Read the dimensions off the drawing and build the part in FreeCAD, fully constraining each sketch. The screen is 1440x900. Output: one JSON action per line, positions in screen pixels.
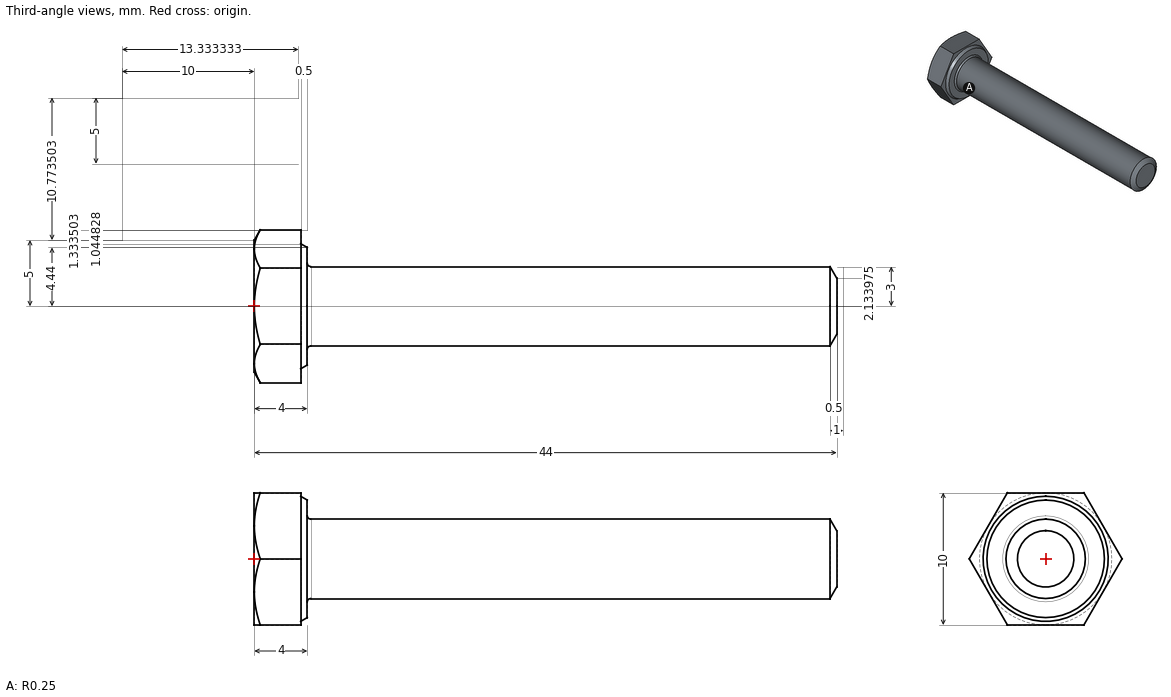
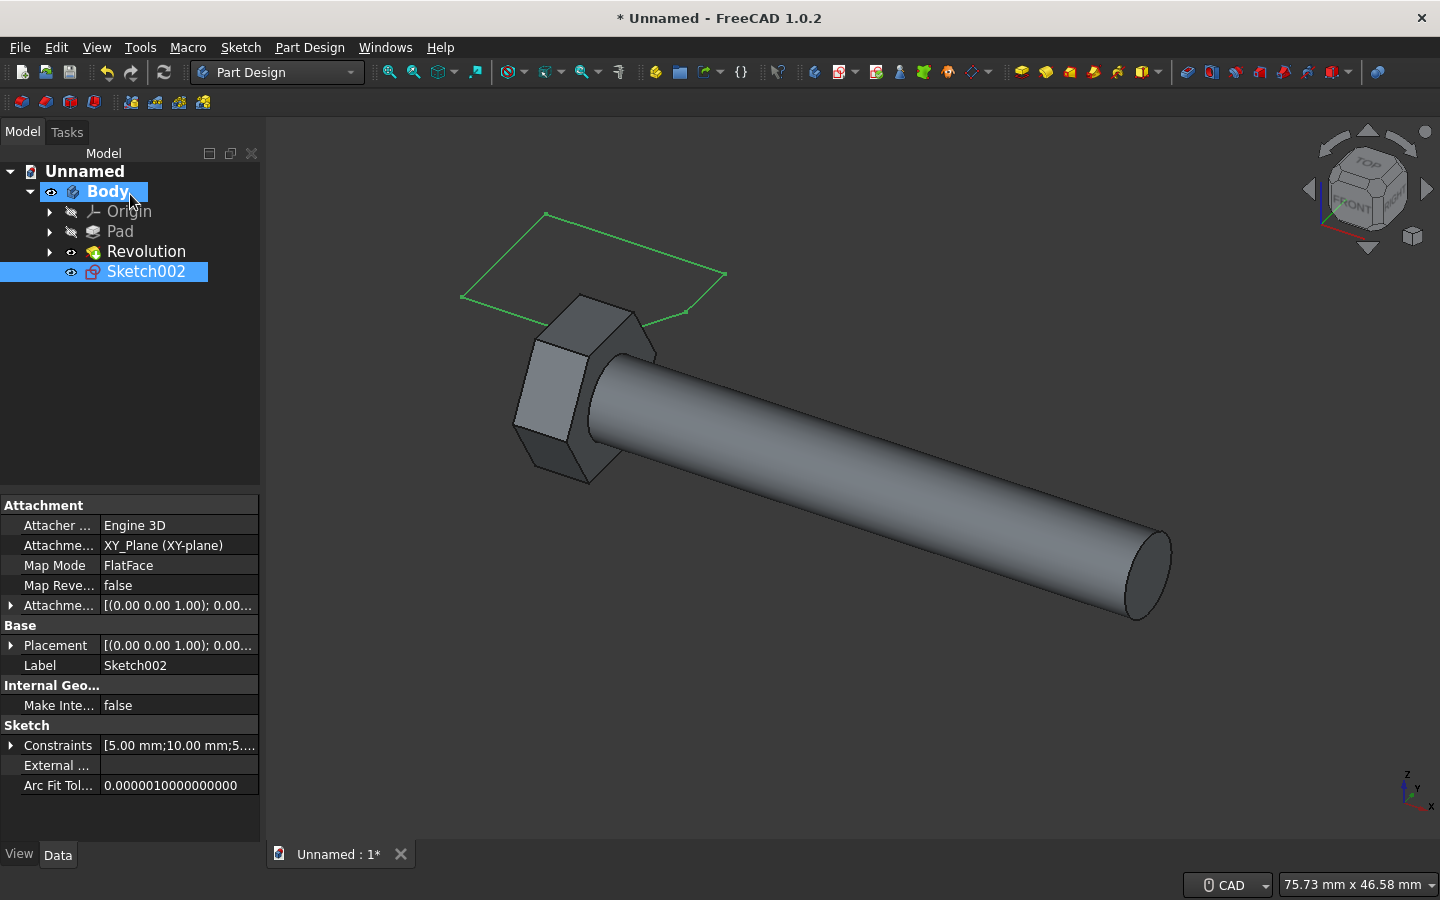
{"action": "left_click", "coordinate": [1236, 72]}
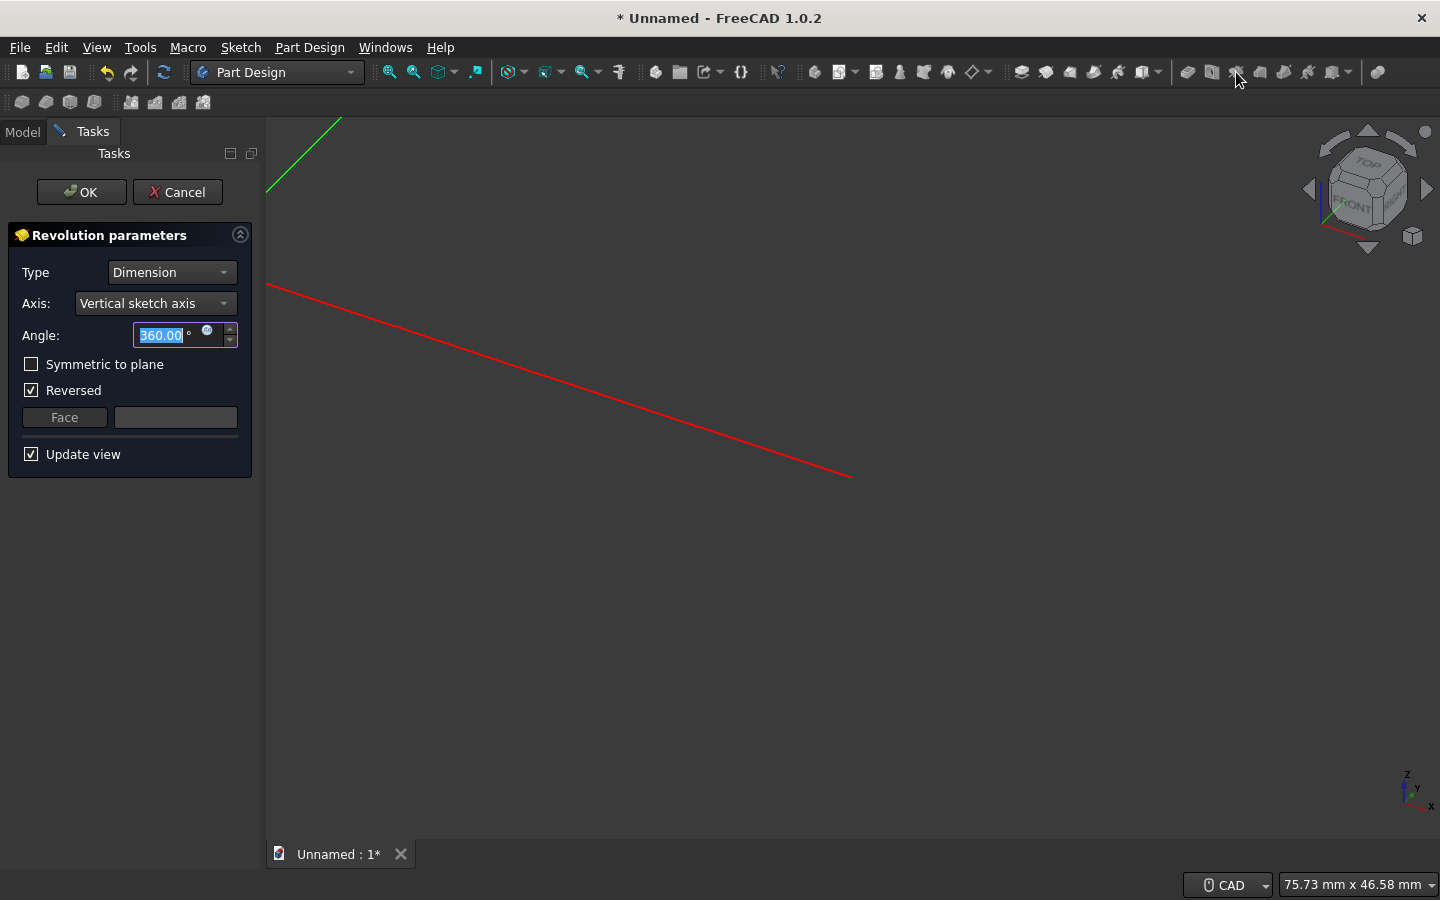
{"action": "left_click", "coordinate": [156, 304]}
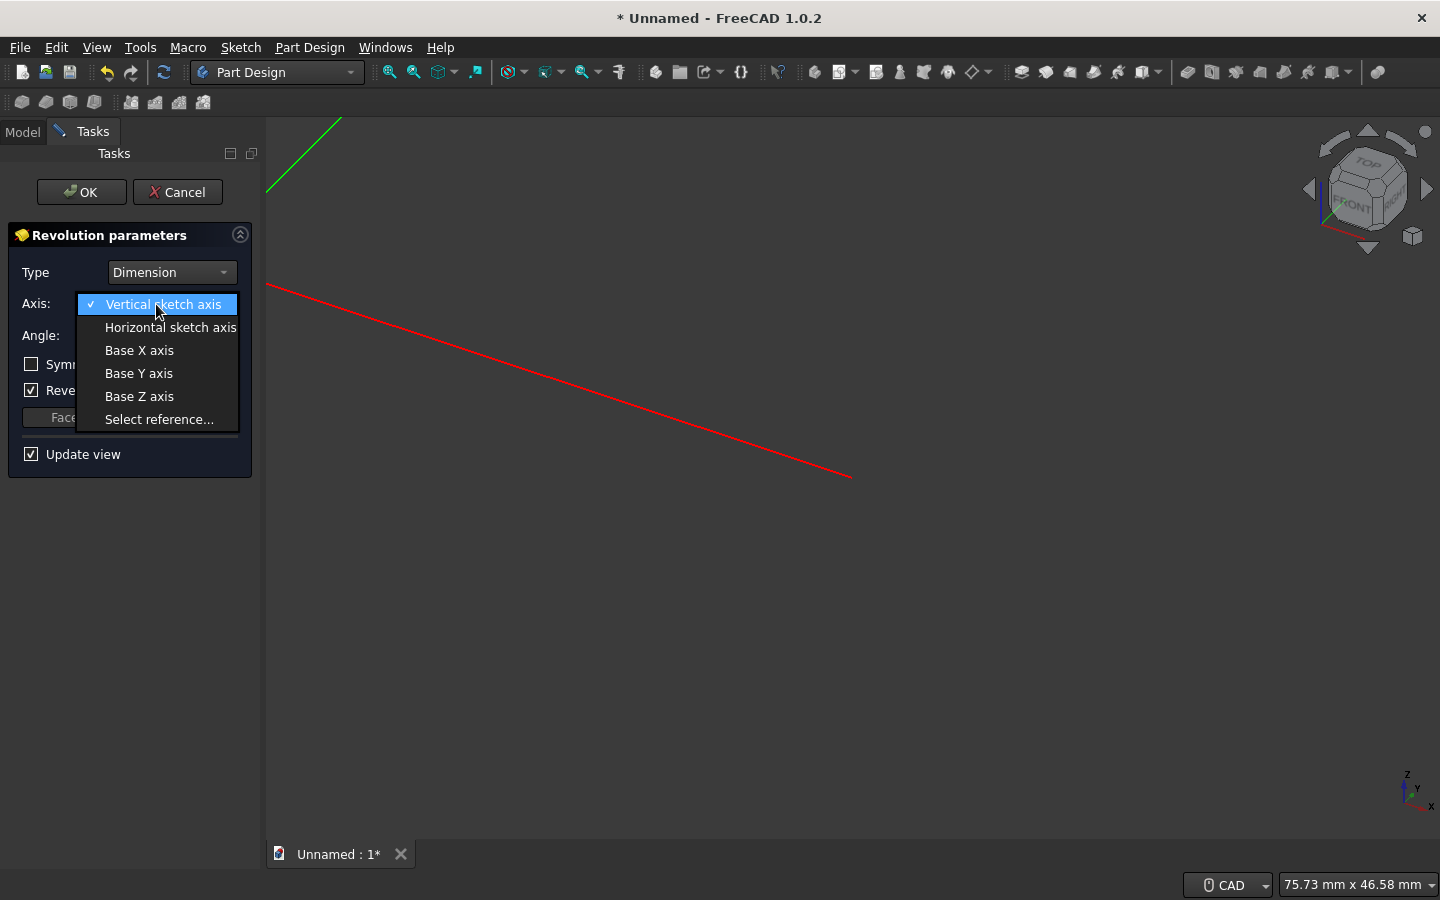
{"action": "left_click", "coordinate": [156, 328]}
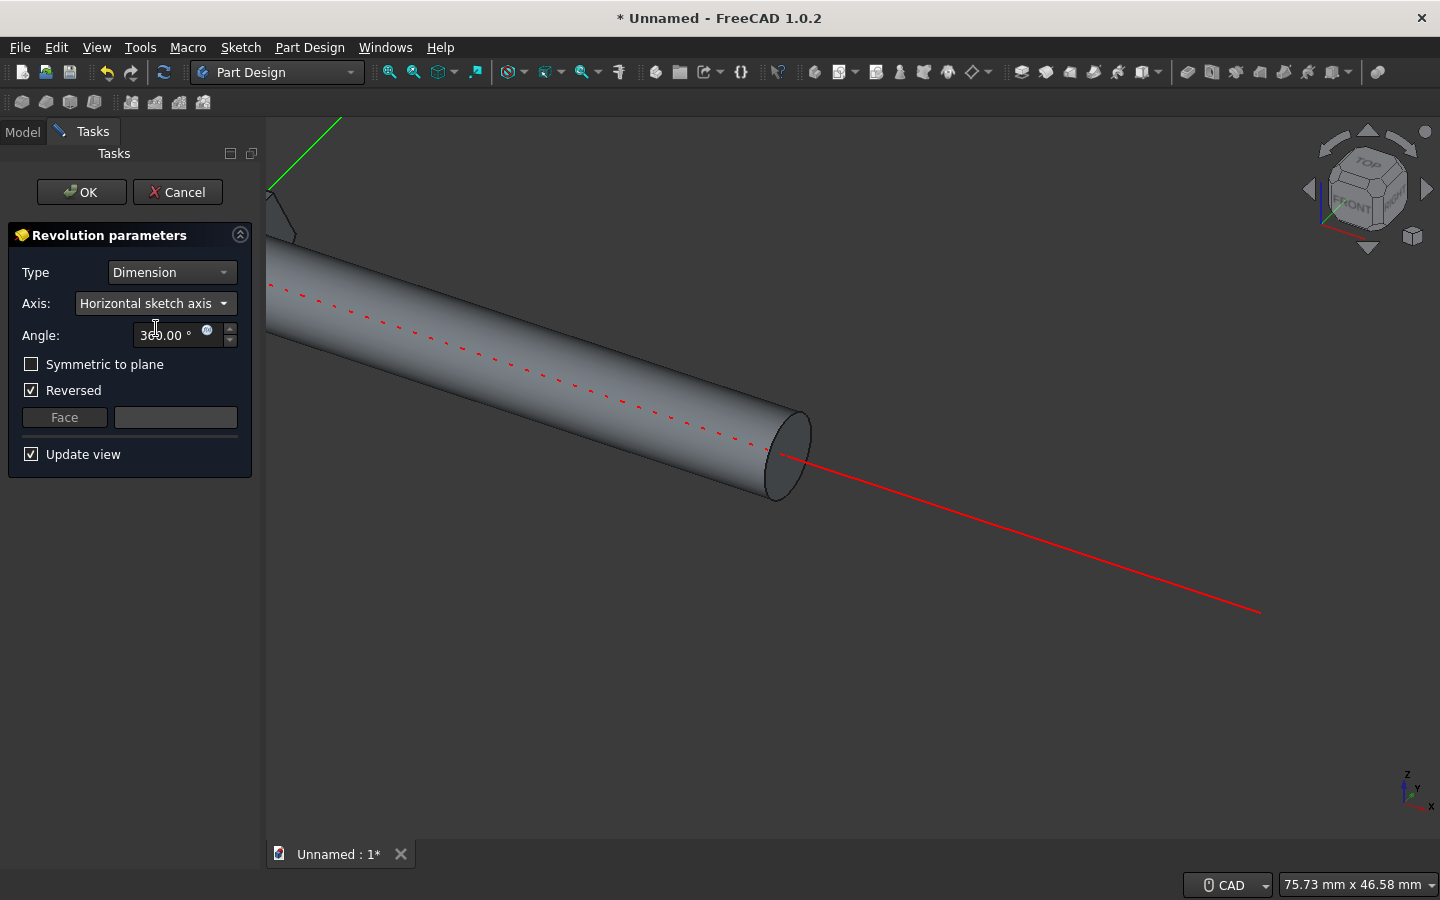
{"action": "left_click", "coordinate": [82, 192]}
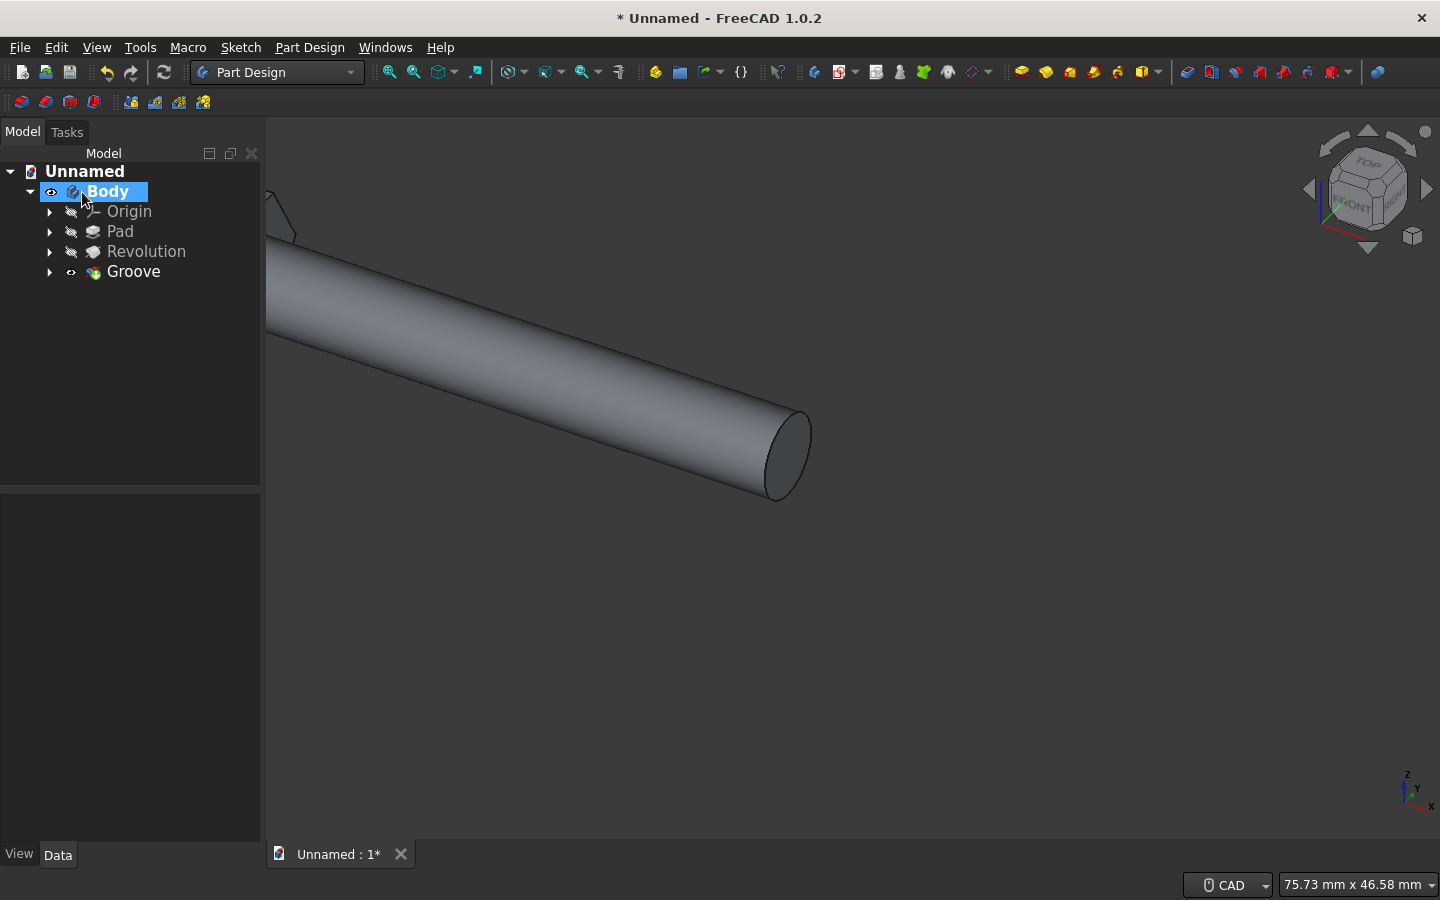
{"action": "left_click", "coordinate": [390, 72]}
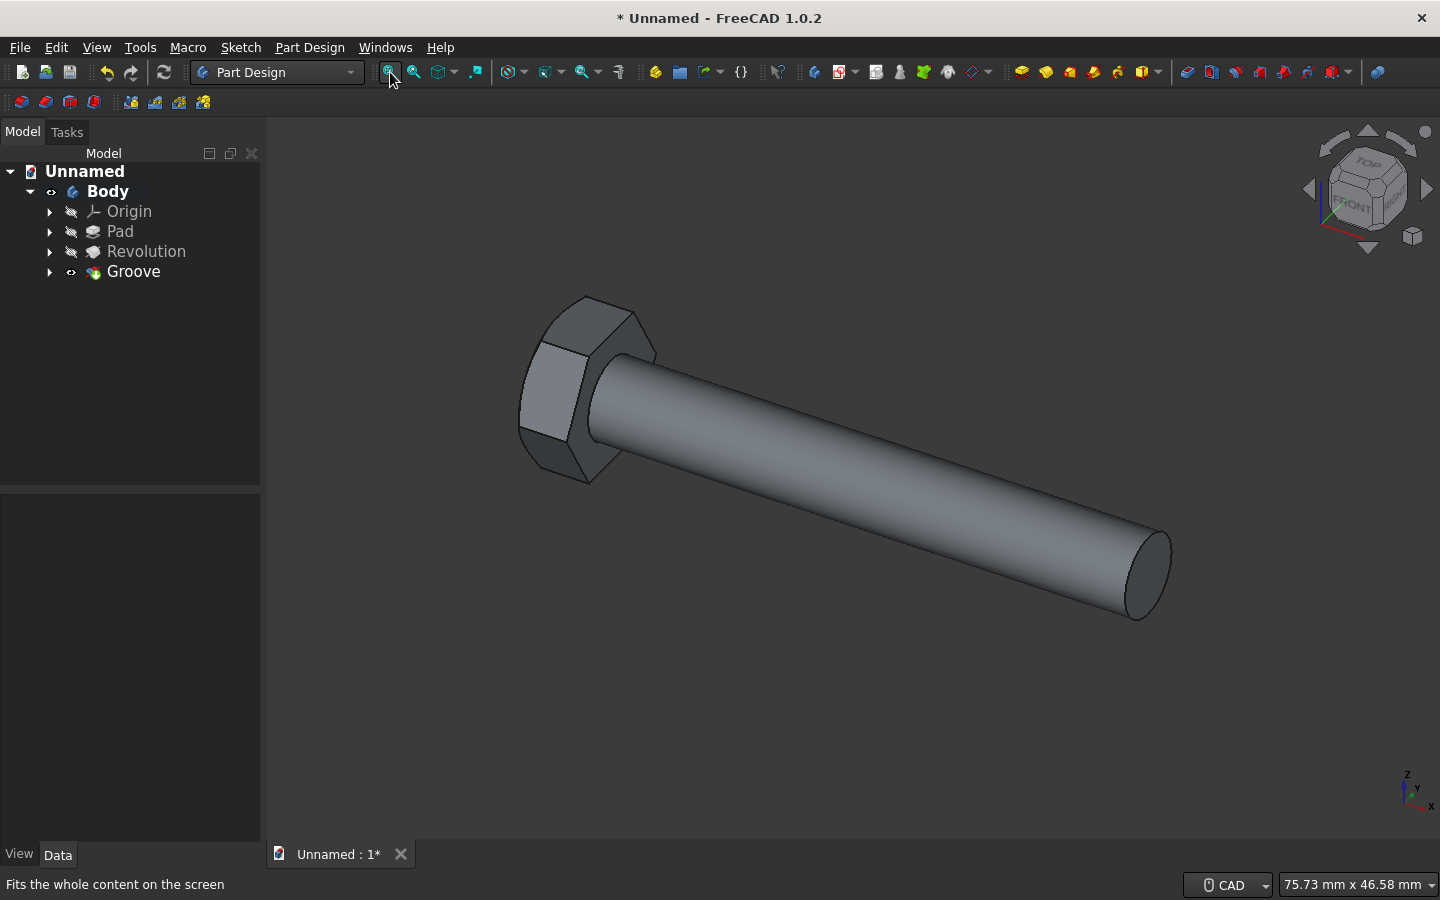
{"action": "left_click", "coordinate": [840, 72]}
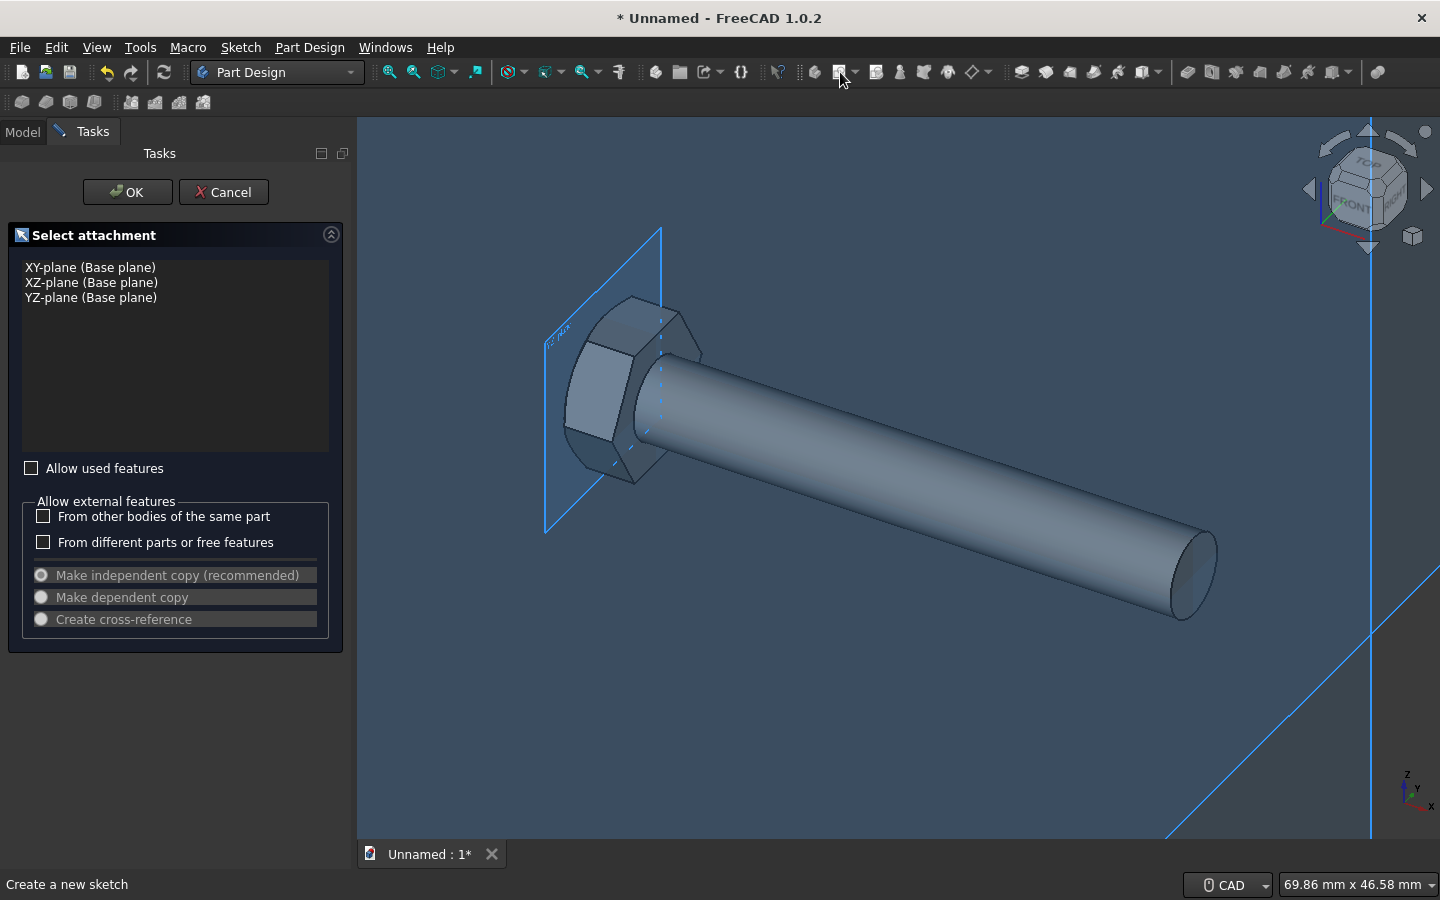
{"action": "left_click", "coordinate": [82, 268]}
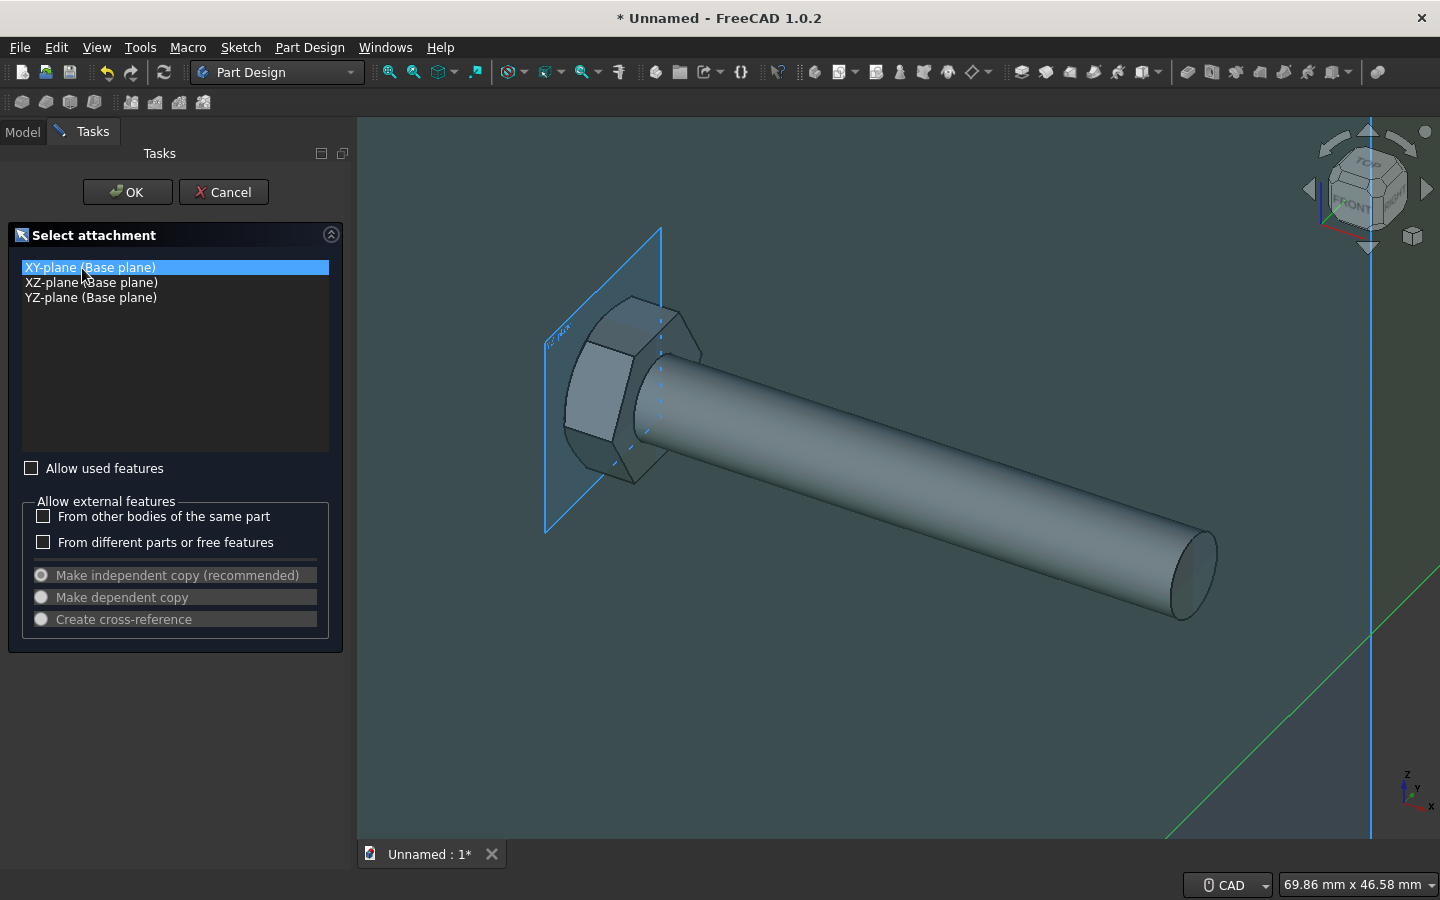
{"action": "left_click", "coordinate": [128, 192]}